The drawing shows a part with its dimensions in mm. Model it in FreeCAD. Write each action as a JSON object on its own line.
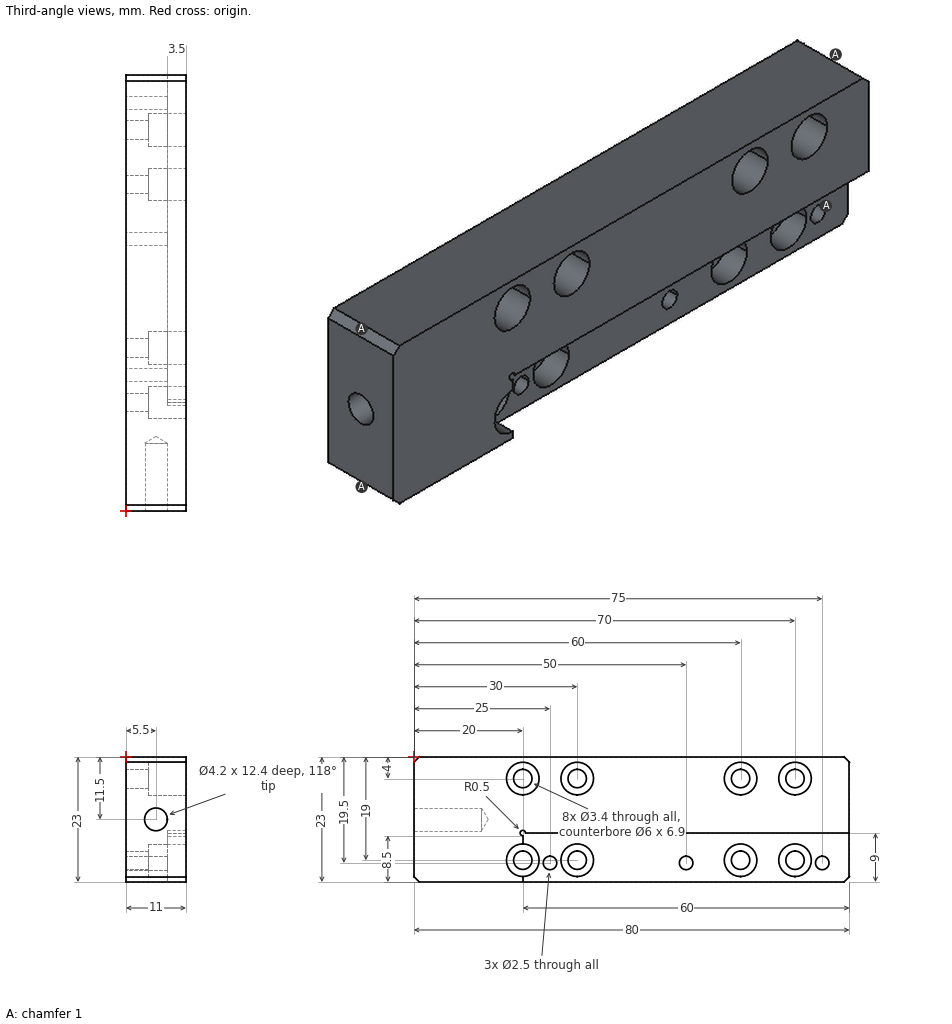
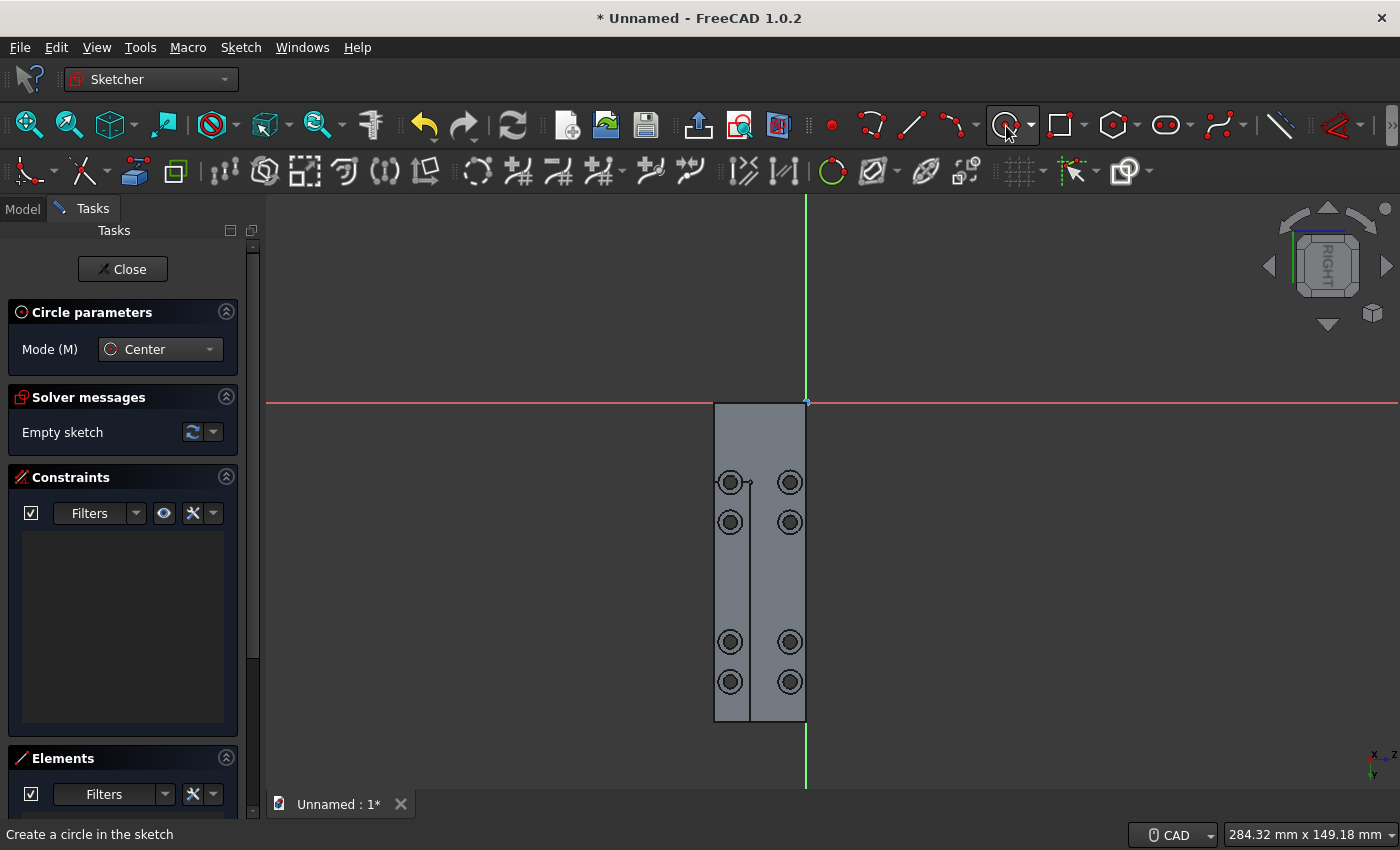
{"action": "scroll", "coordinate": [728, 502], "scroll_direction": "up", "scroll_amount": 8}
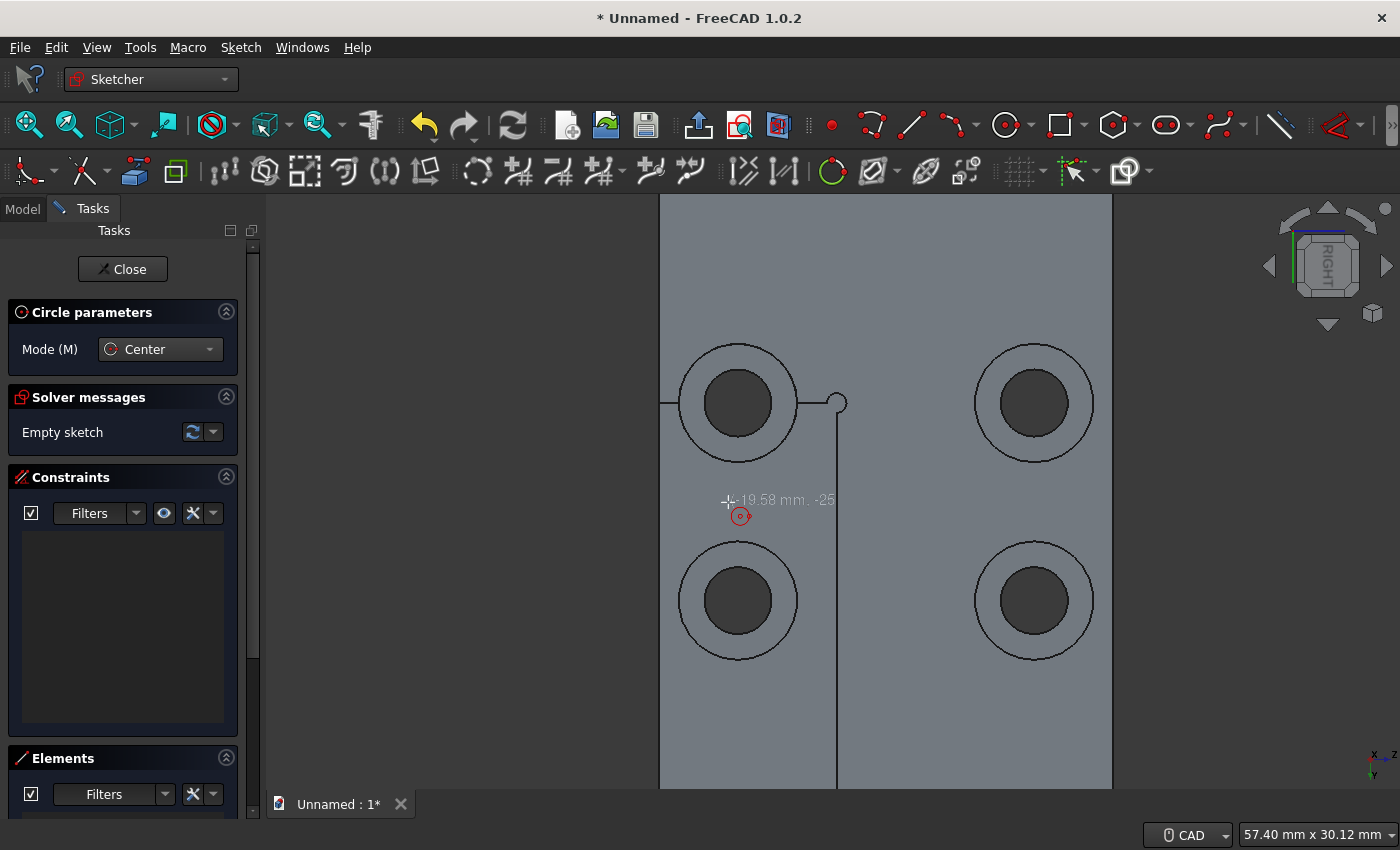
{"action": "scroll", "coordinate": [717, 403], "scroll_direction": "down", "scroll_amount": 7}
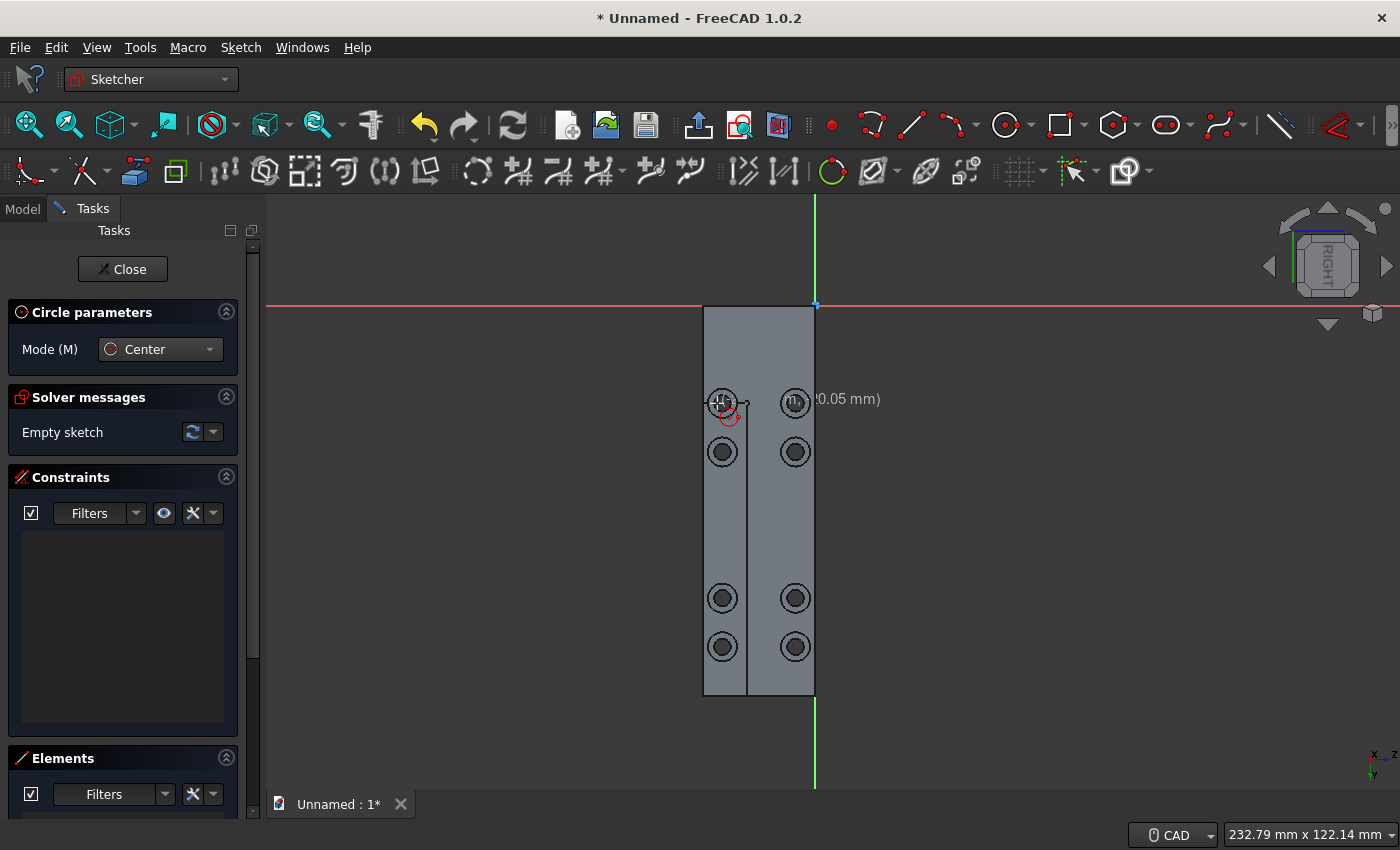
{"action": "left_click", "coordinate": [720, 428]}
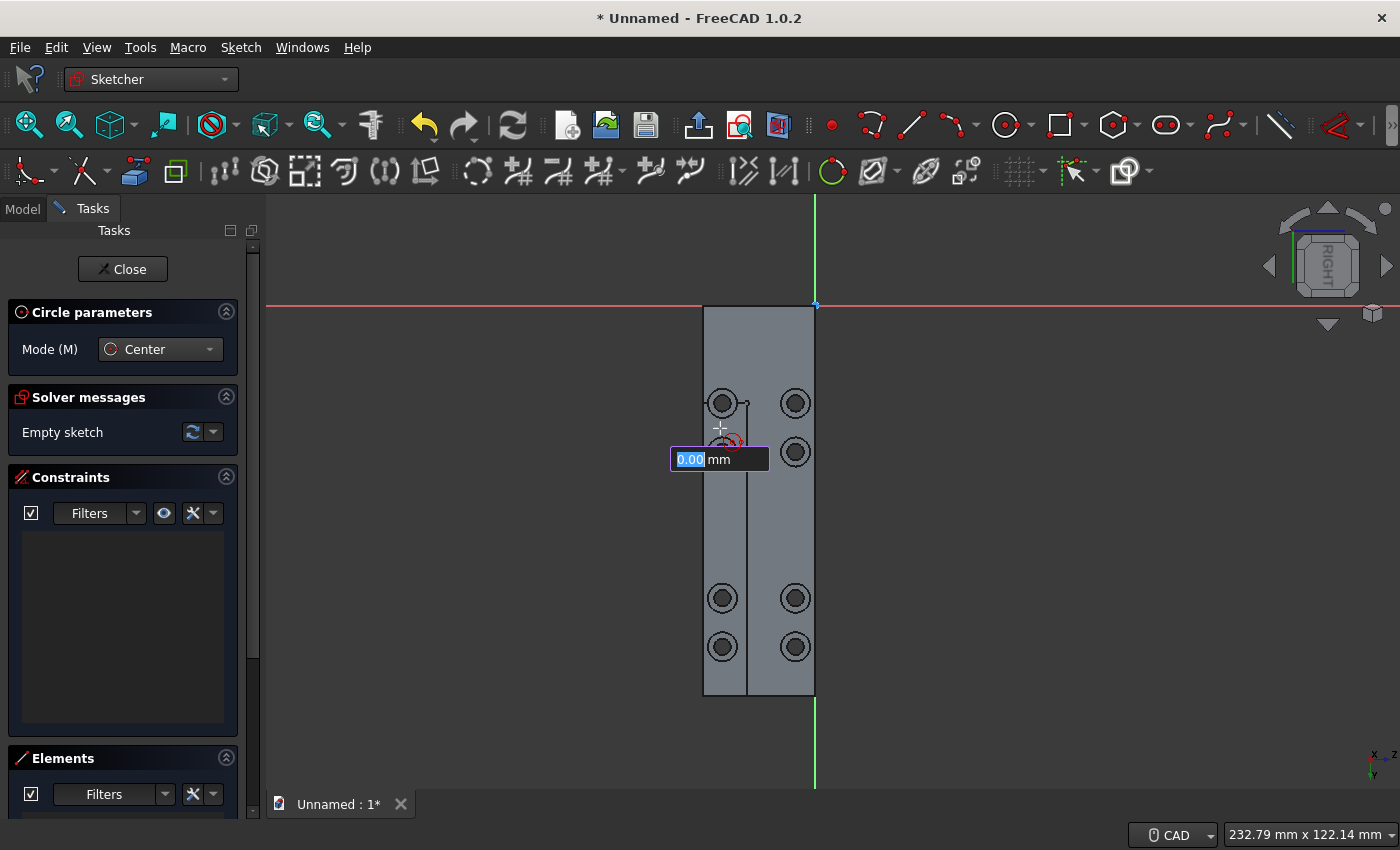
{"action": "scroll", "coordinate": [724, 423], "scroll_direction": "up", "scroll_amount": 5}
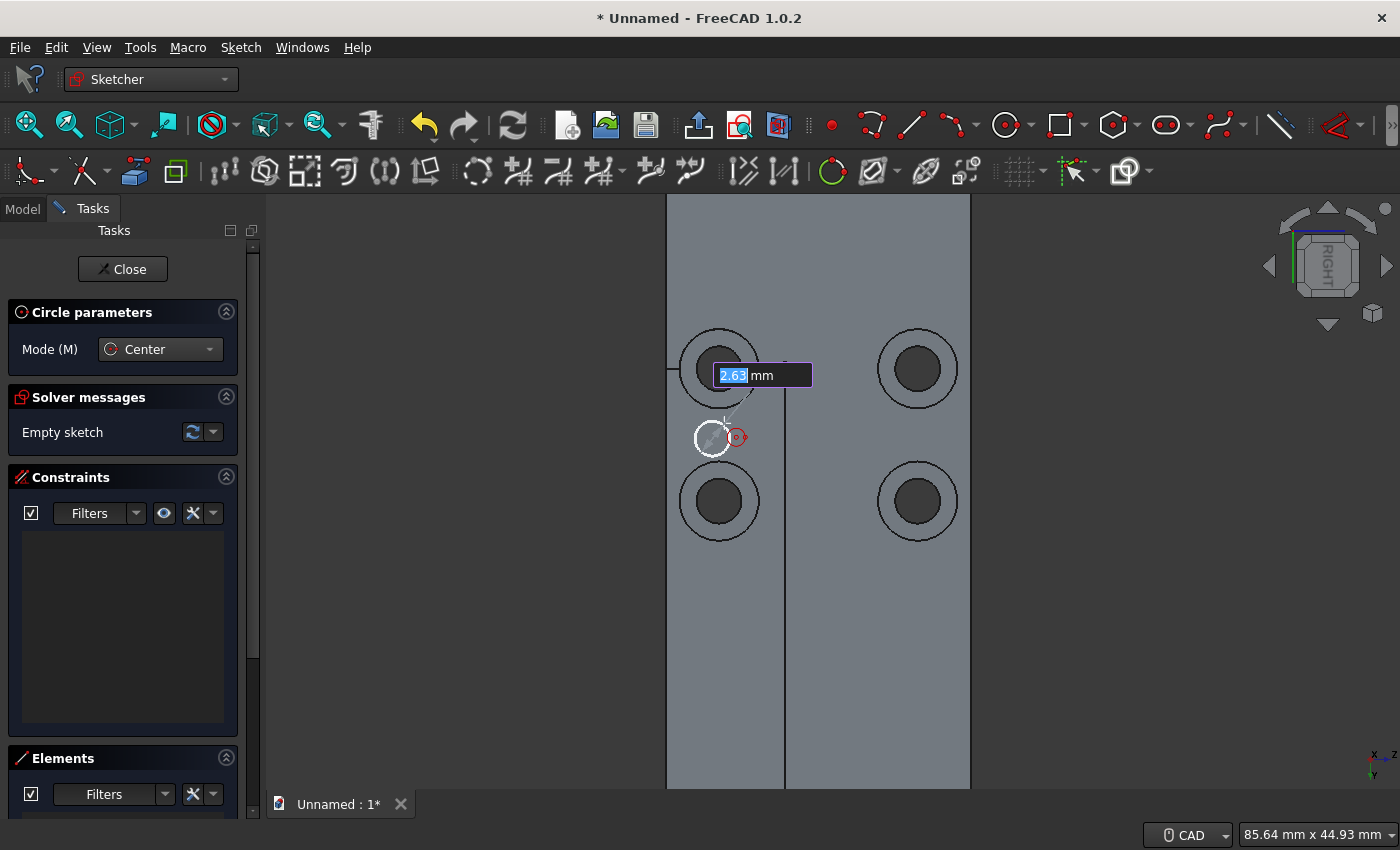
{"action": "left_click", "coordinate": [724, 423]}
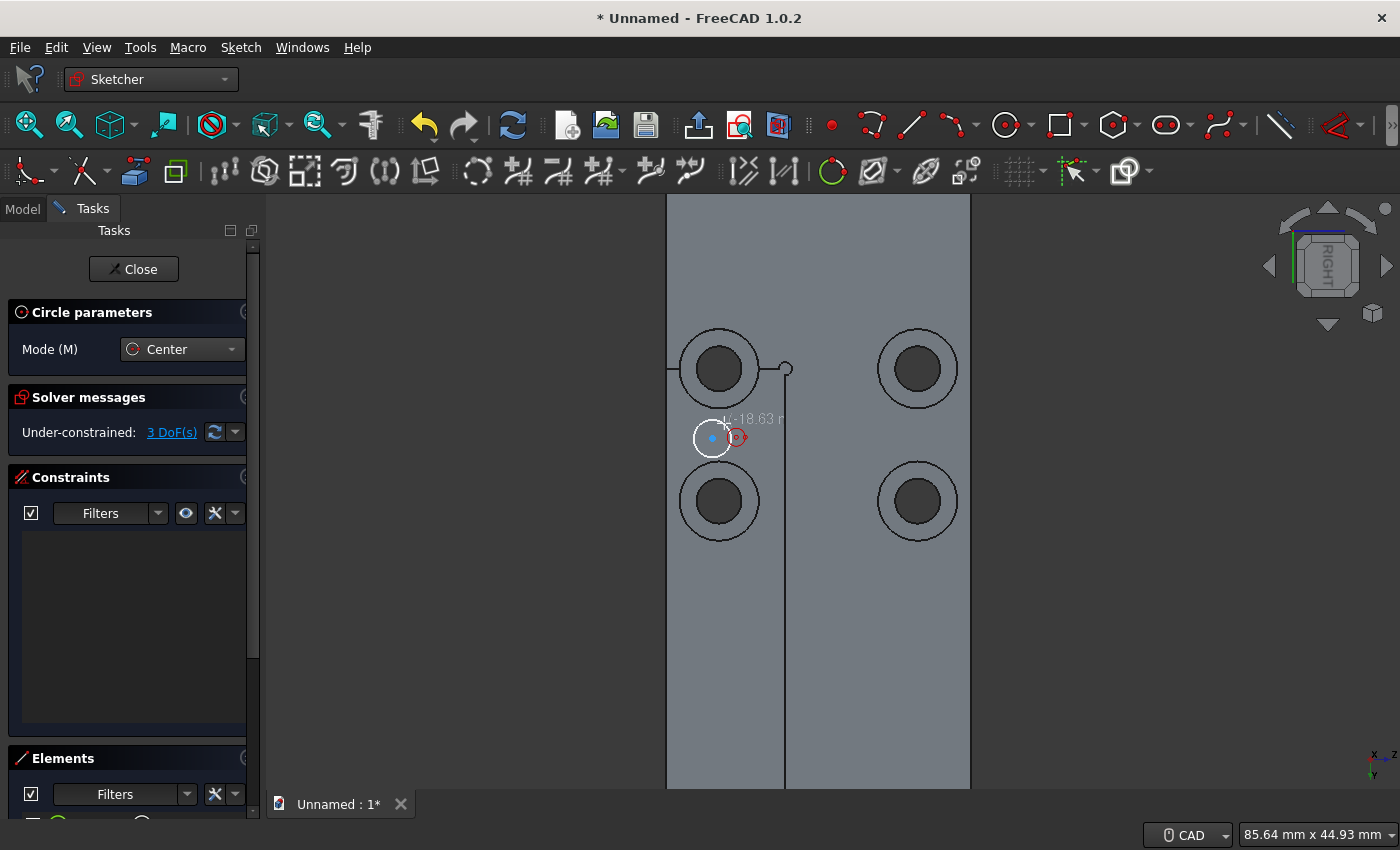
{"action": "scroll", "coordinate": [724, 423], "scroll_direction": "down", "scroll_amount": 5}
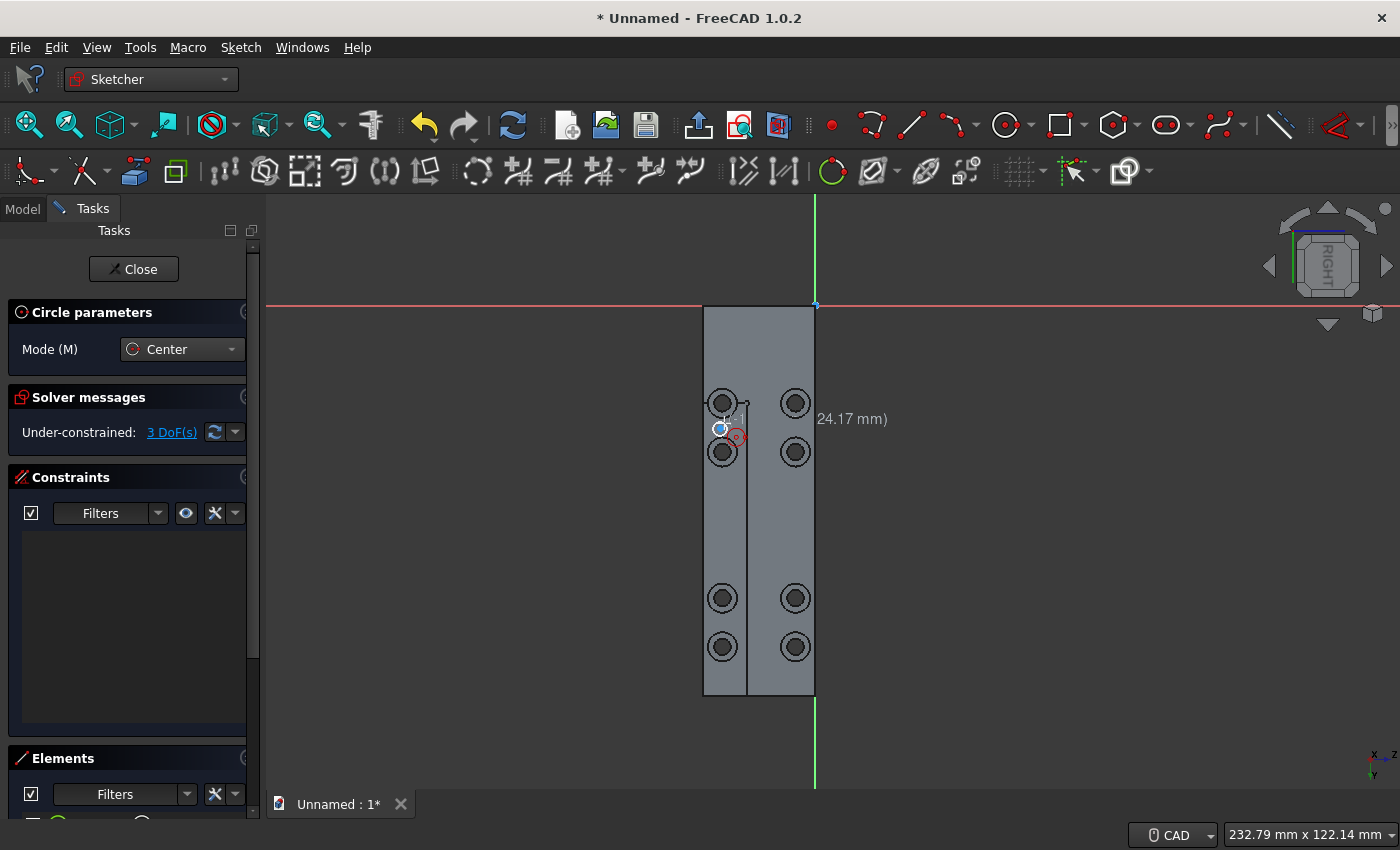
{"action": "scroll", "coordinate": [720, 549], "scroll_direction": "up", "scroll_amount": 7}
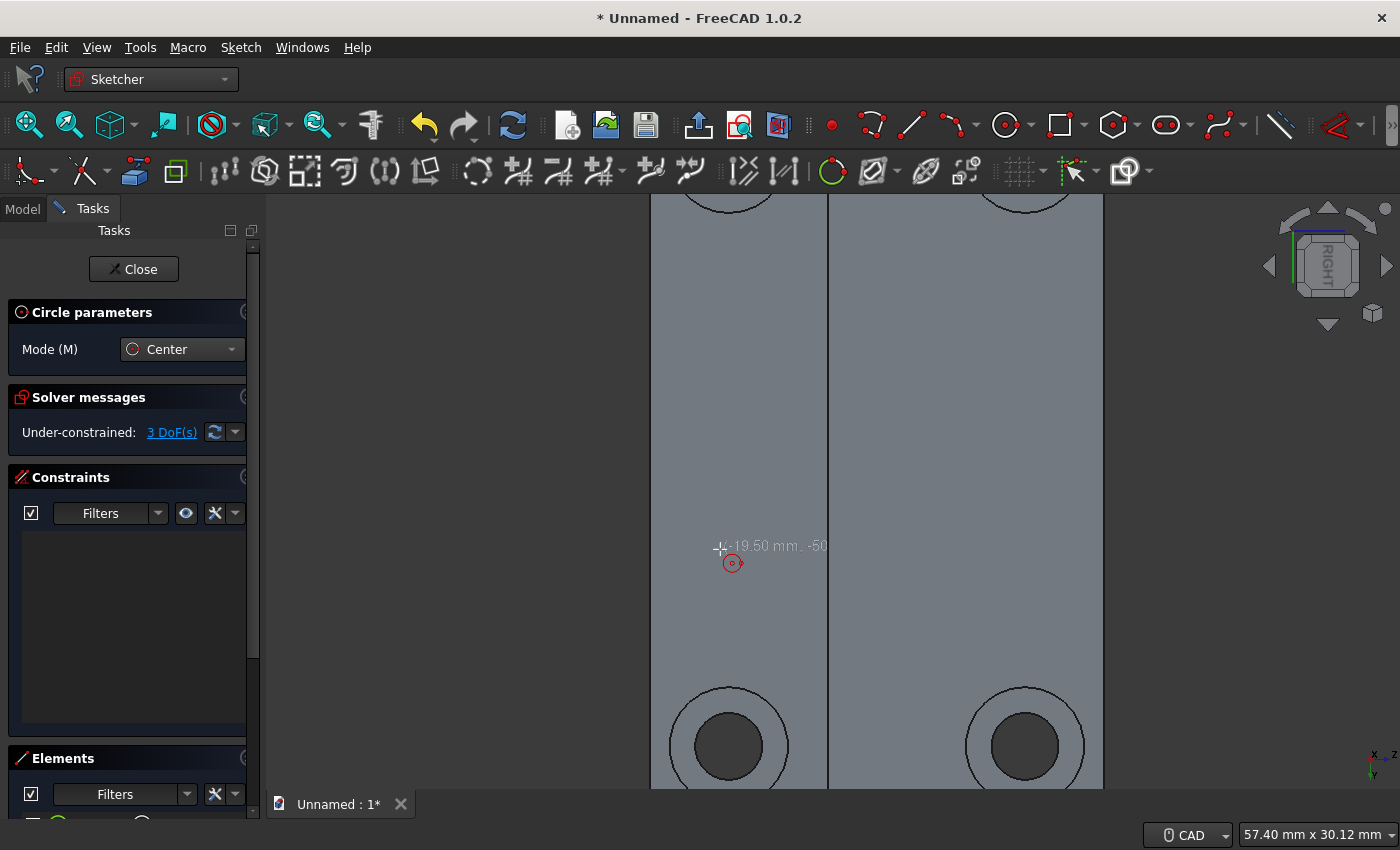
{"action": "scroll", "coordinate": [720, 550], "scroll_direction": "down", "scroll_amount": 7}